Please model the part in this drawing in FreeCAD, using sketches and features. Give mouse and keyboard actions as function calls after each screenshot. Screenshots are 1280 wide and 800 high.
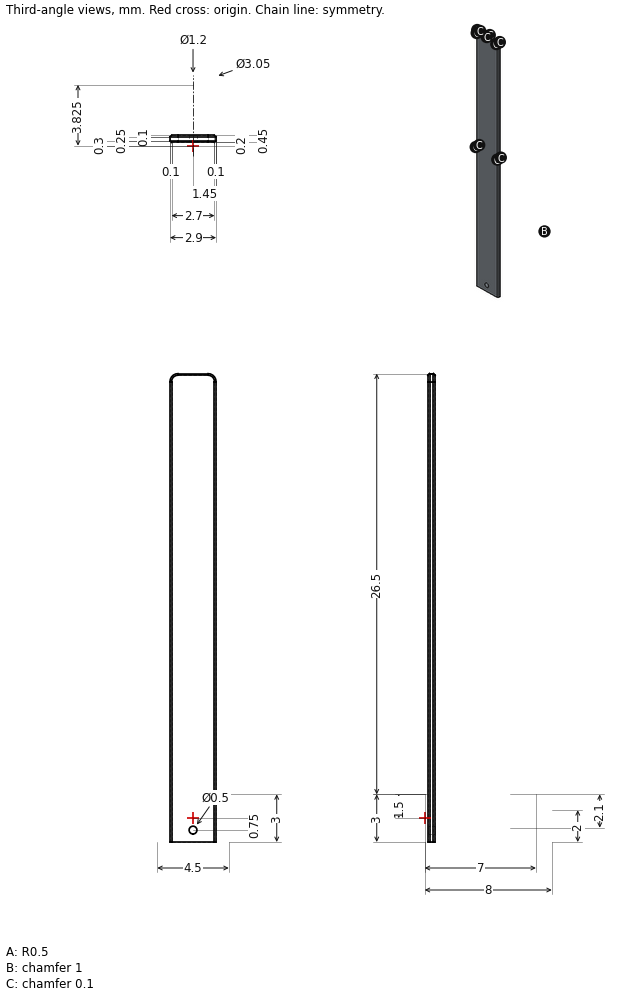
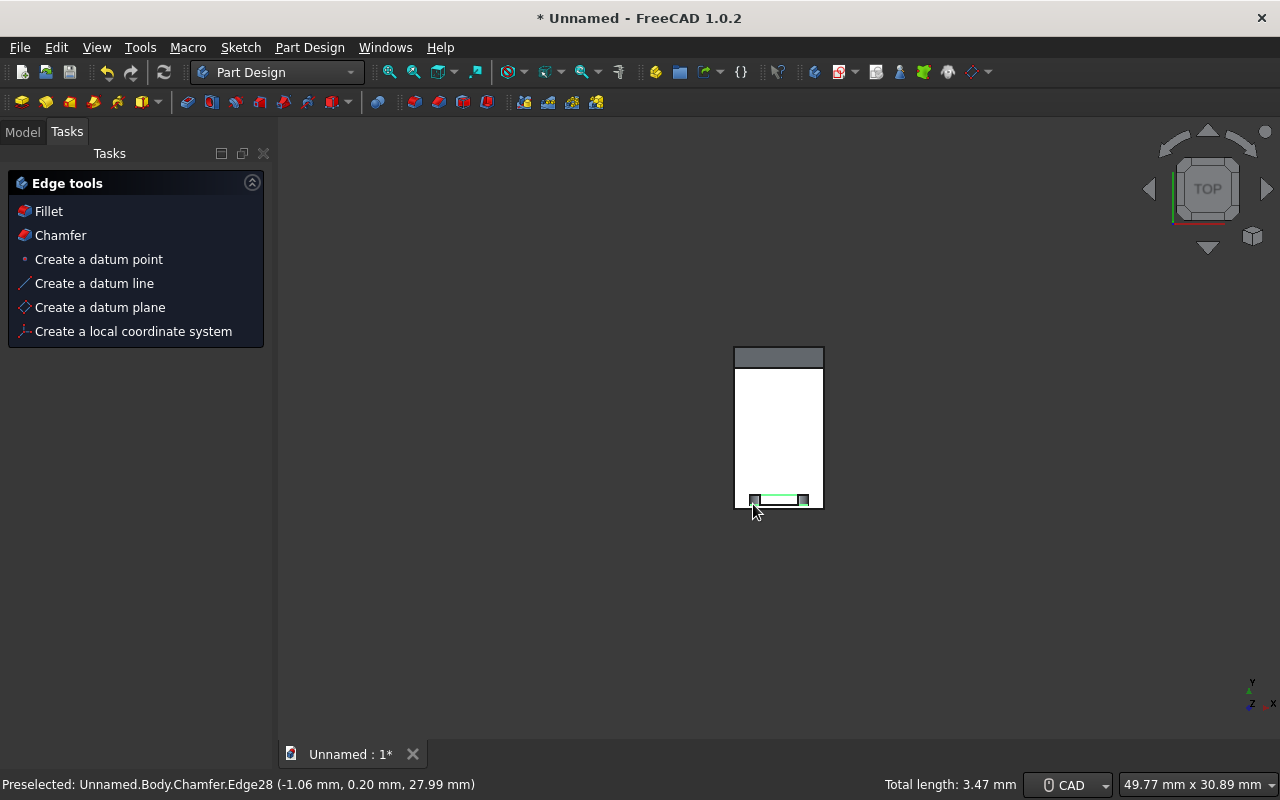
click(805, 494, ctrl)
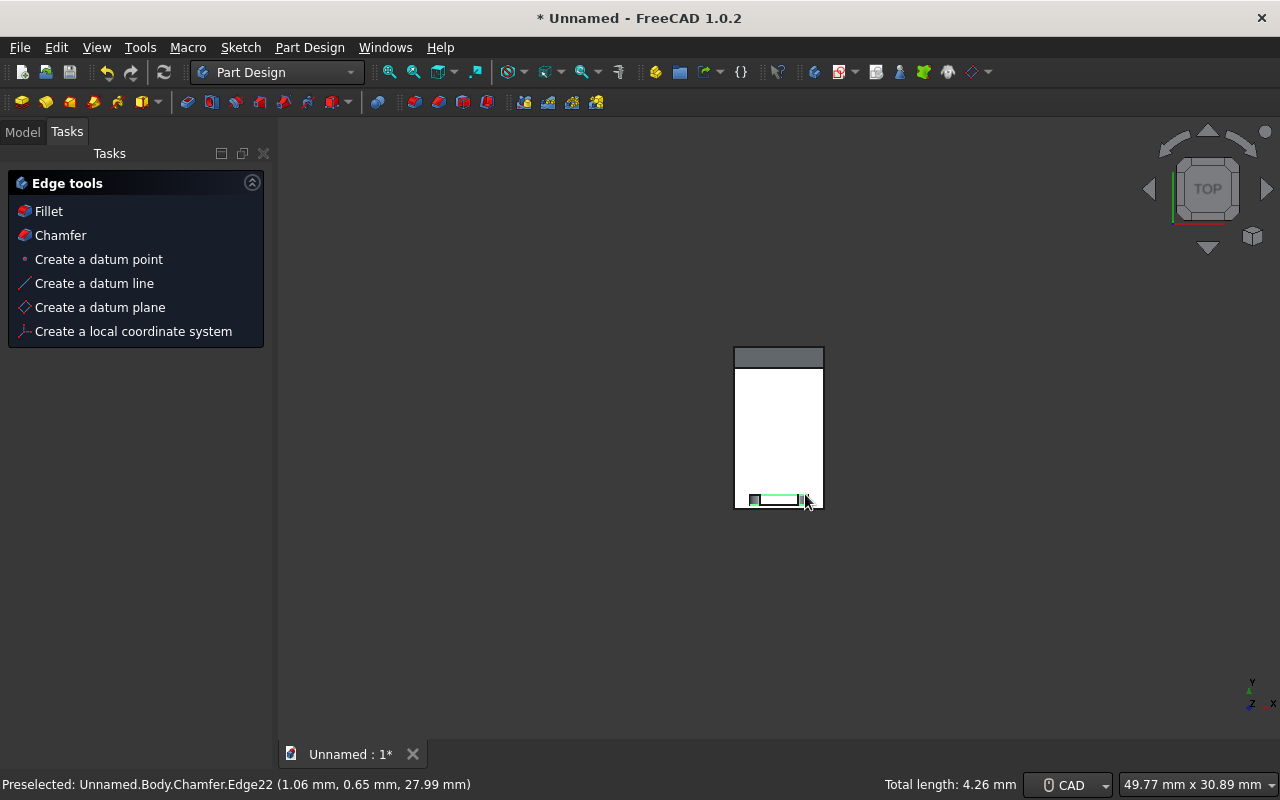
click(753, 494, ctrl)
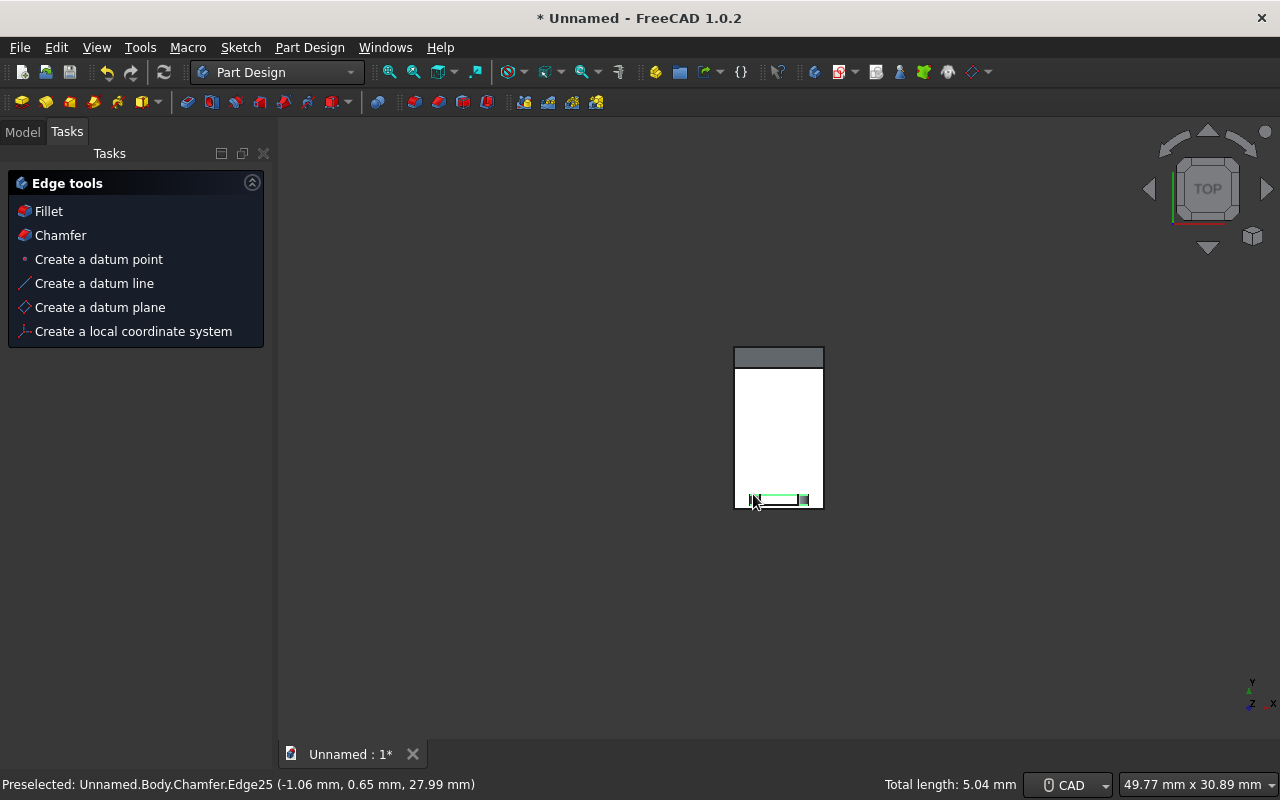
key(0)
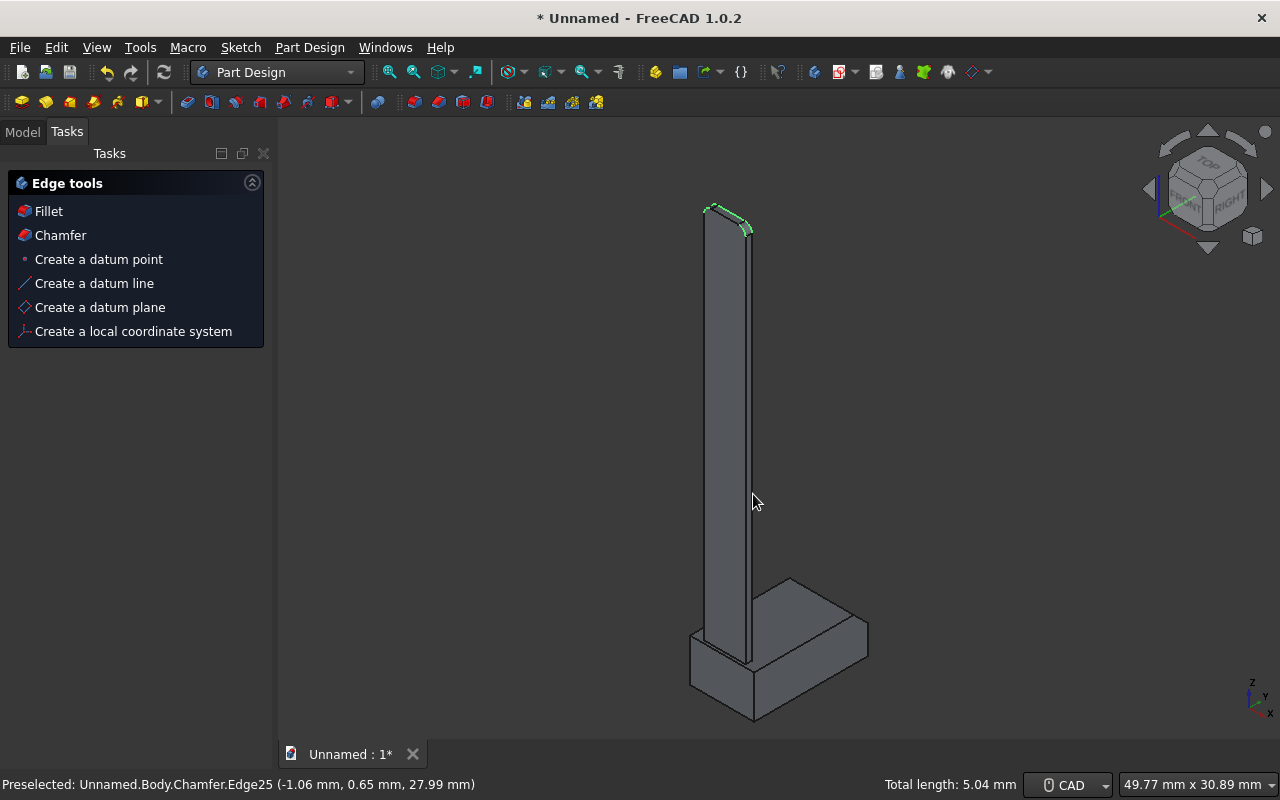
click(725, 216, ctrl)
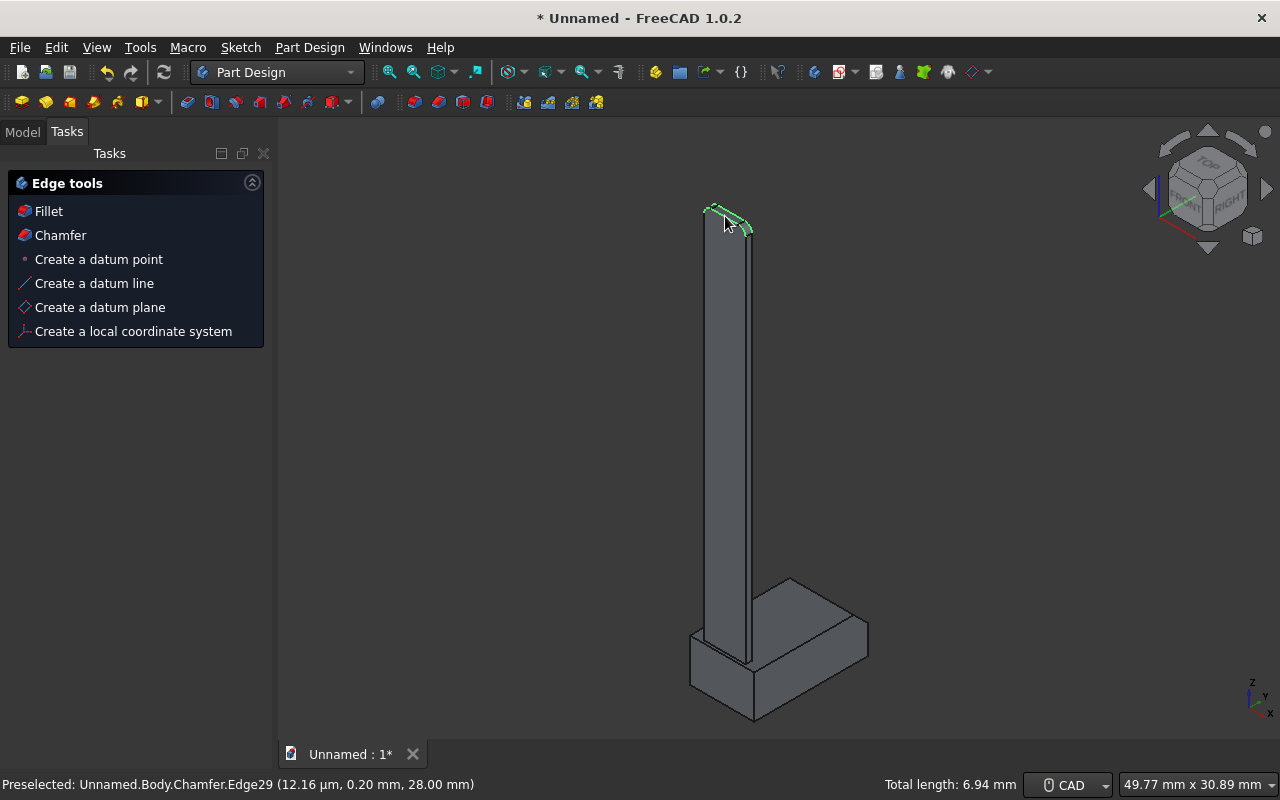
click(746, 450, ctrl)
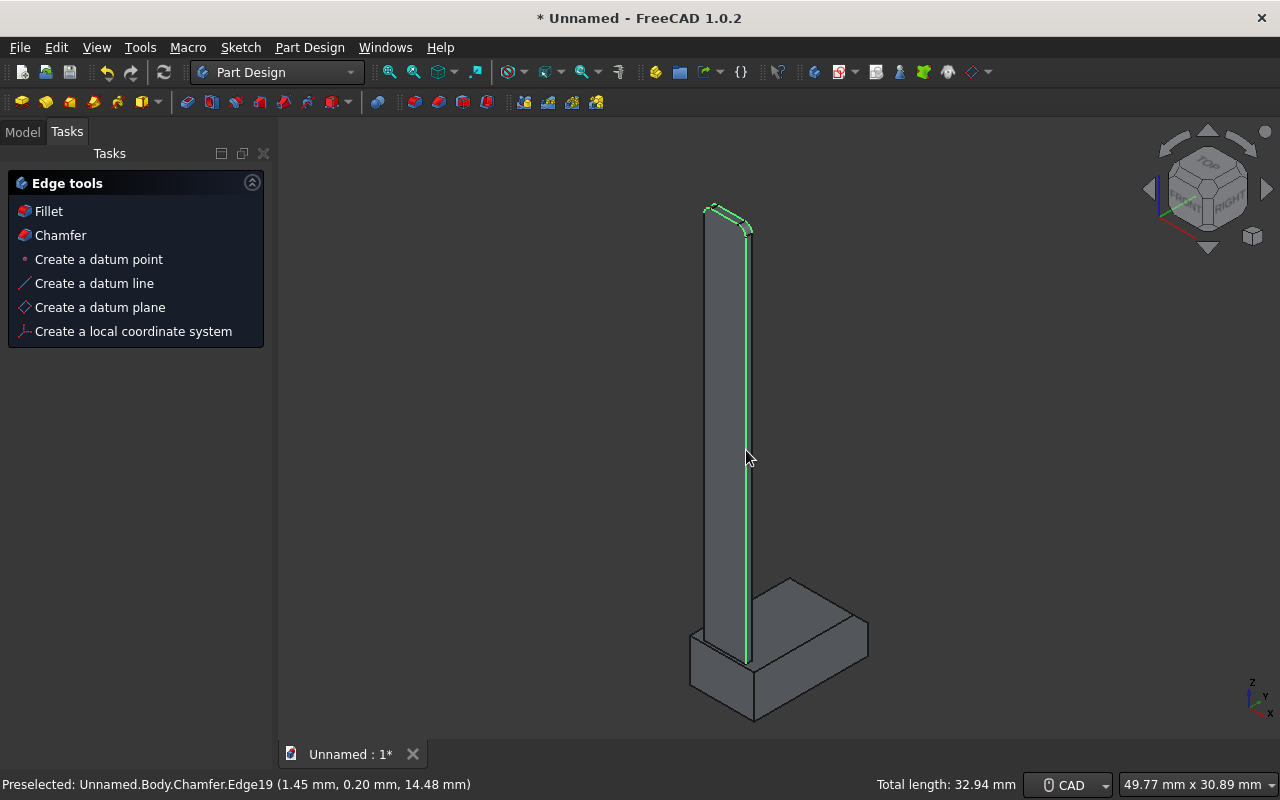
key(2)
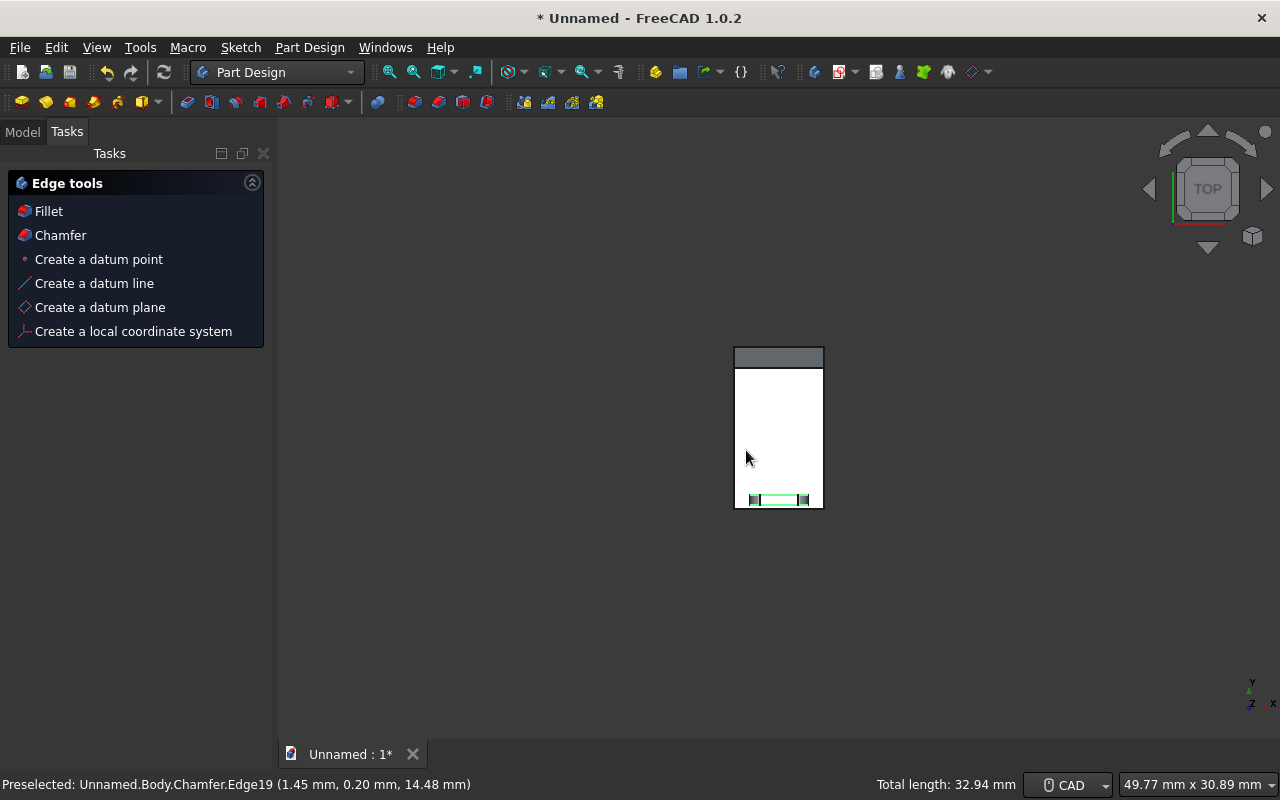
key(v)
key(f)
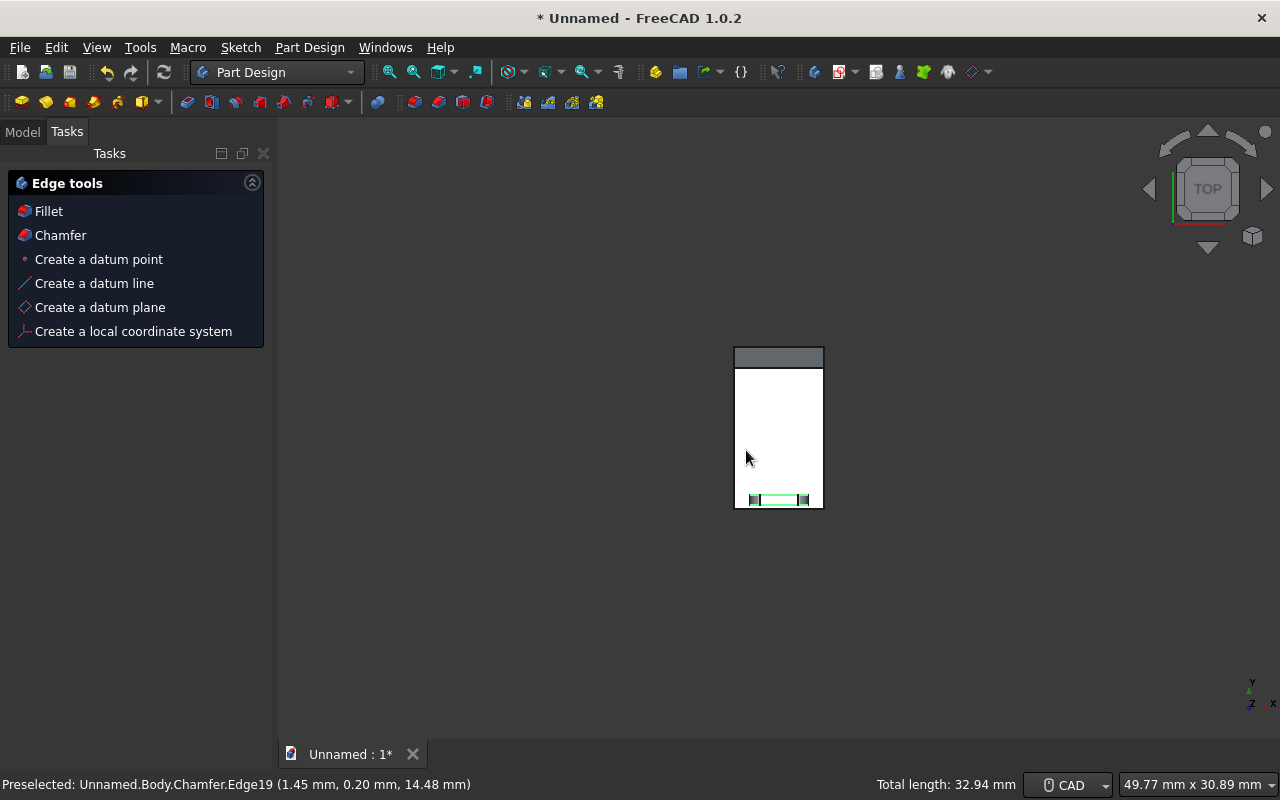
key(1)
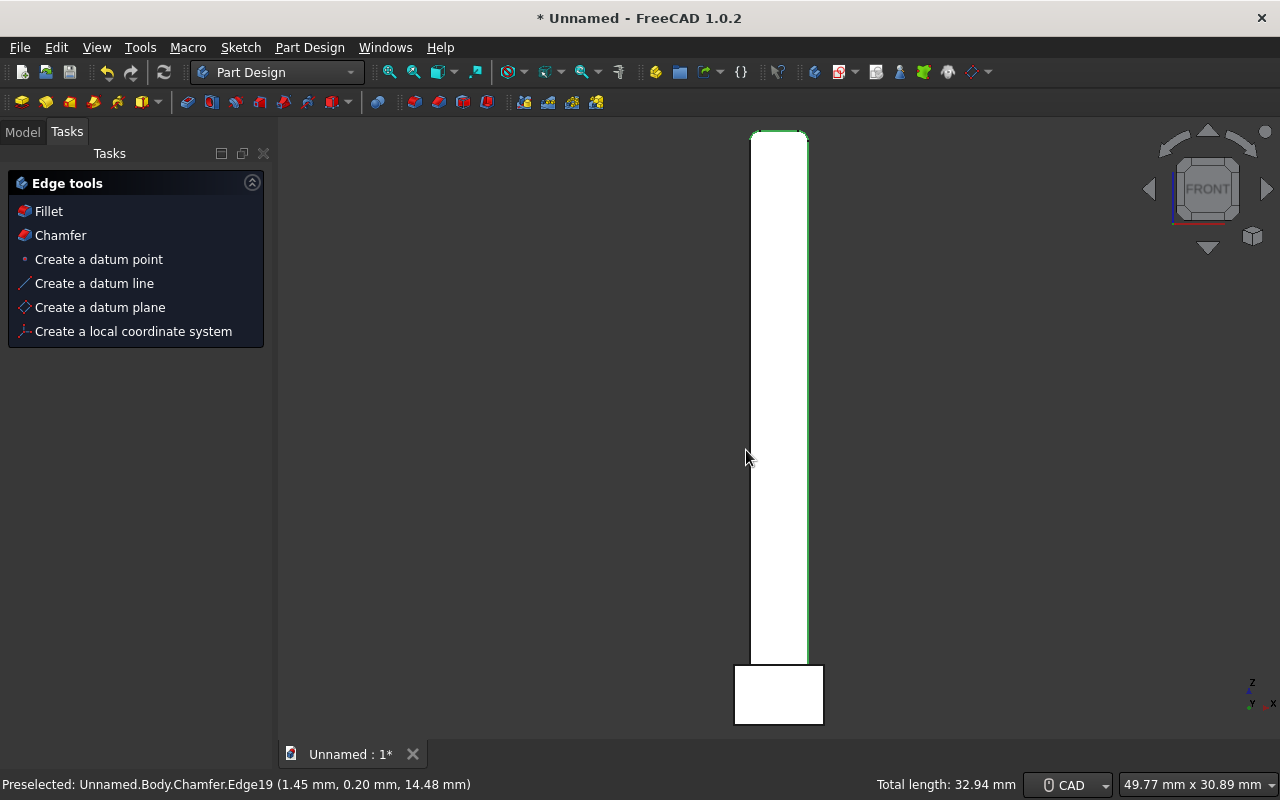
click(750, 402, ctrl)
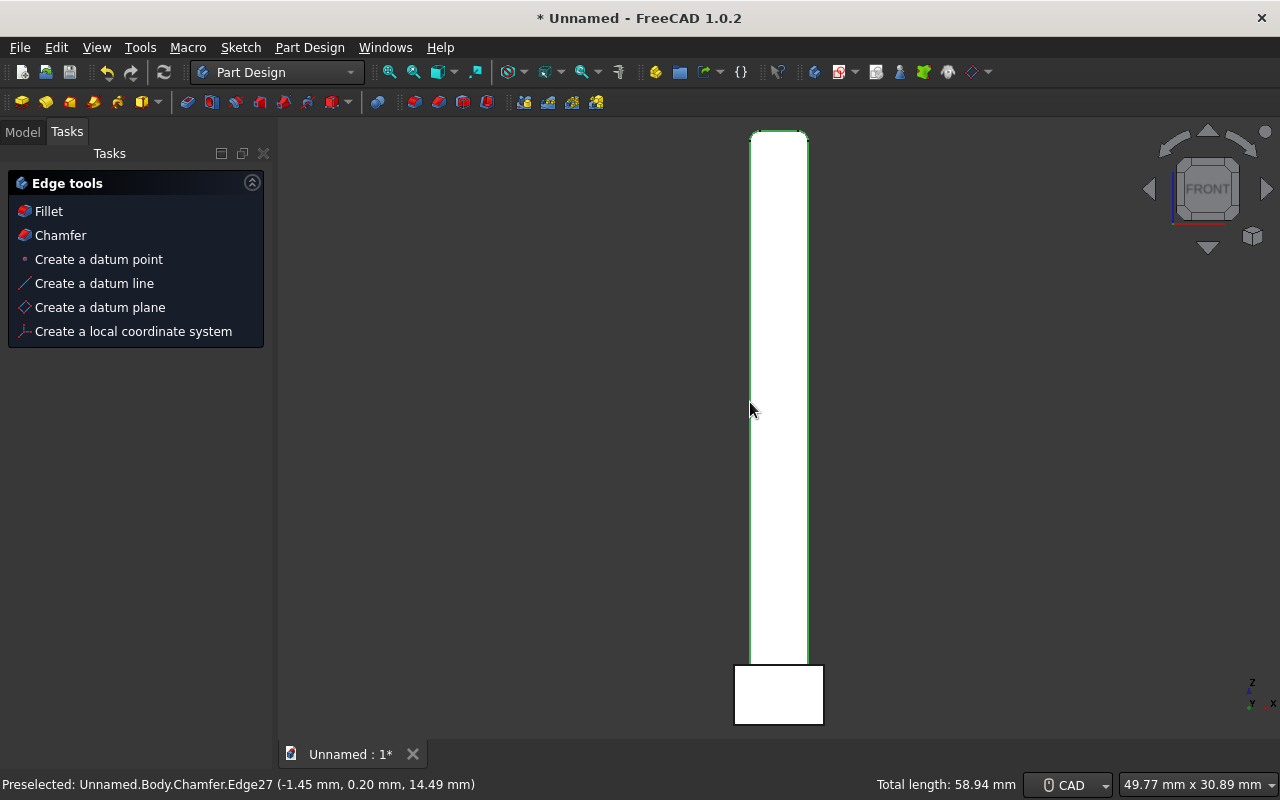
key(3)